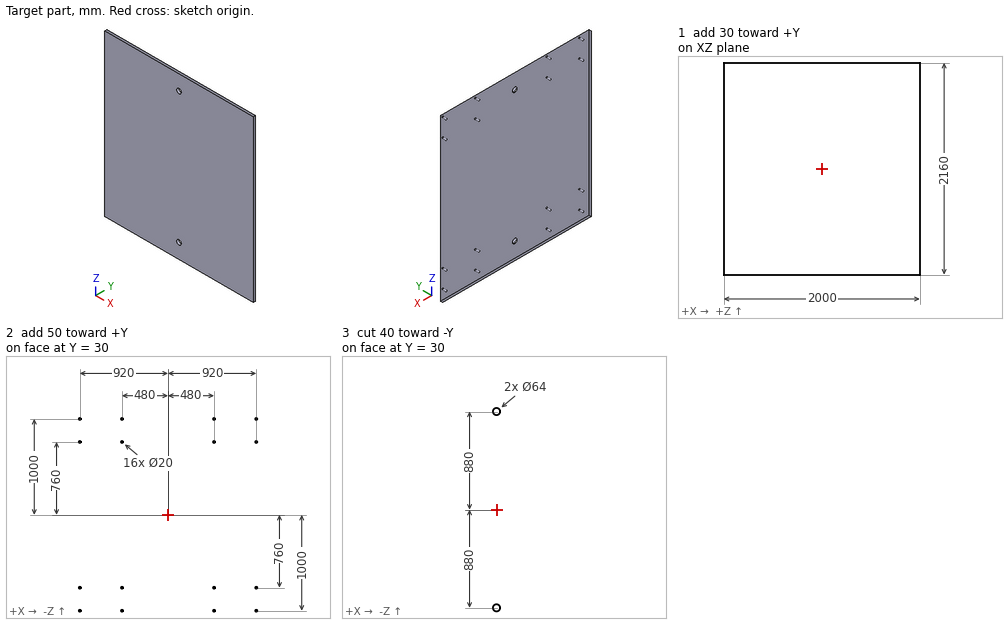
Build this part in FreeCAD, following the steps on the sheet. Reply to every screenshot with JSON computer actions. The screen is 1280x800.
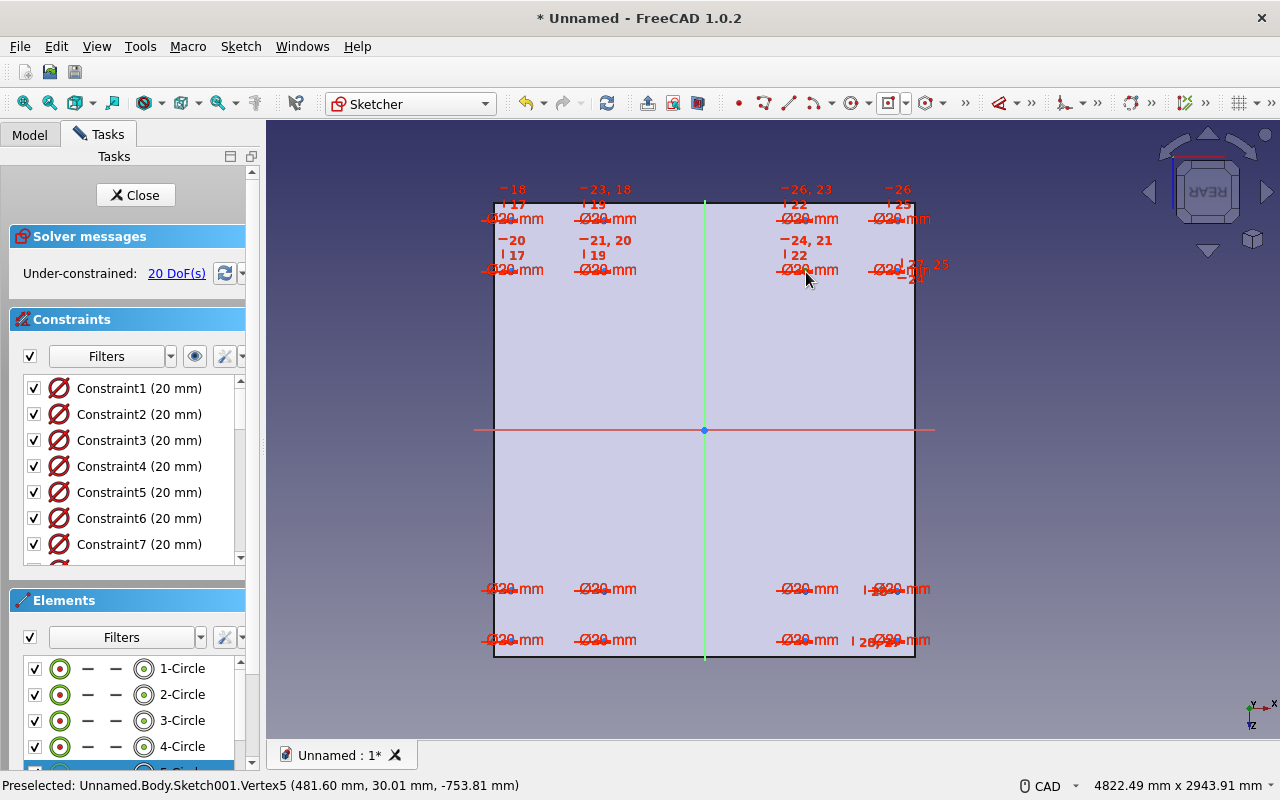
{"action": "left_click", "coordinate": [806, 642]}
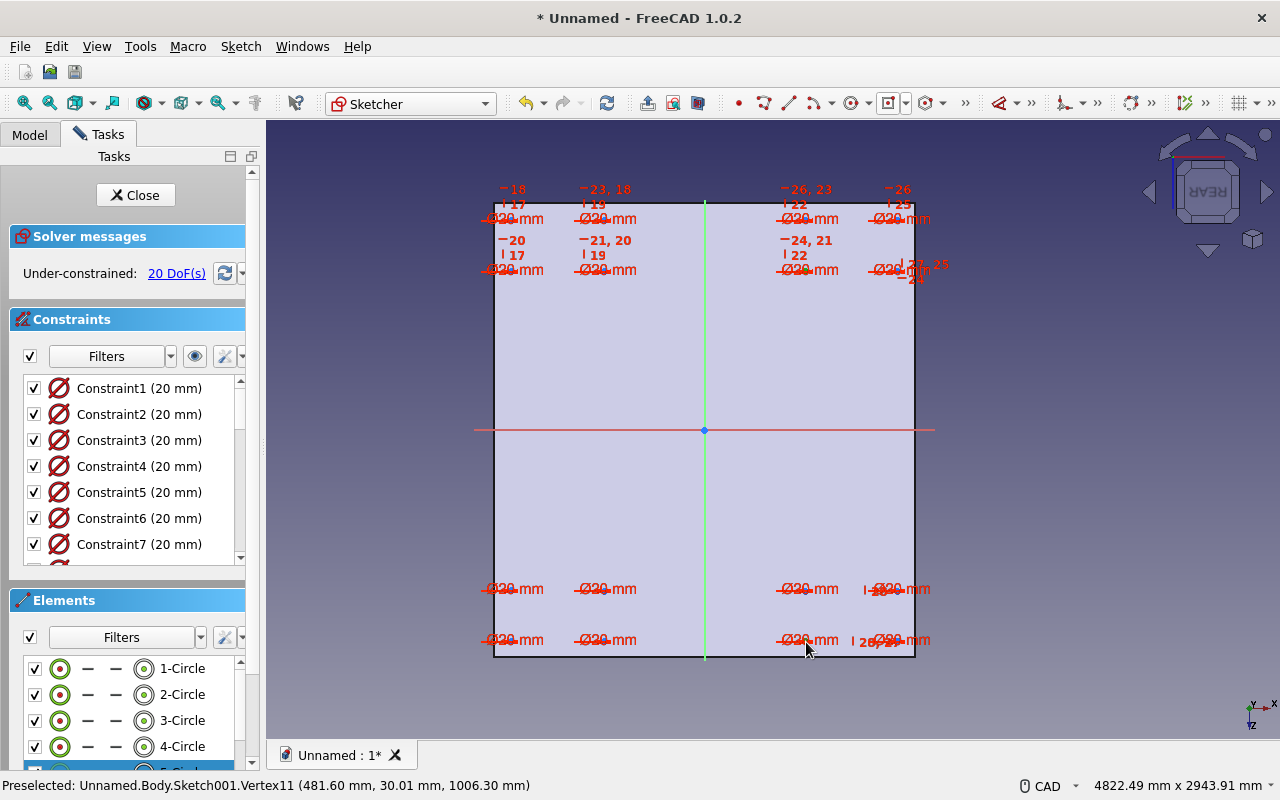
{"action": "key", "text": "v"}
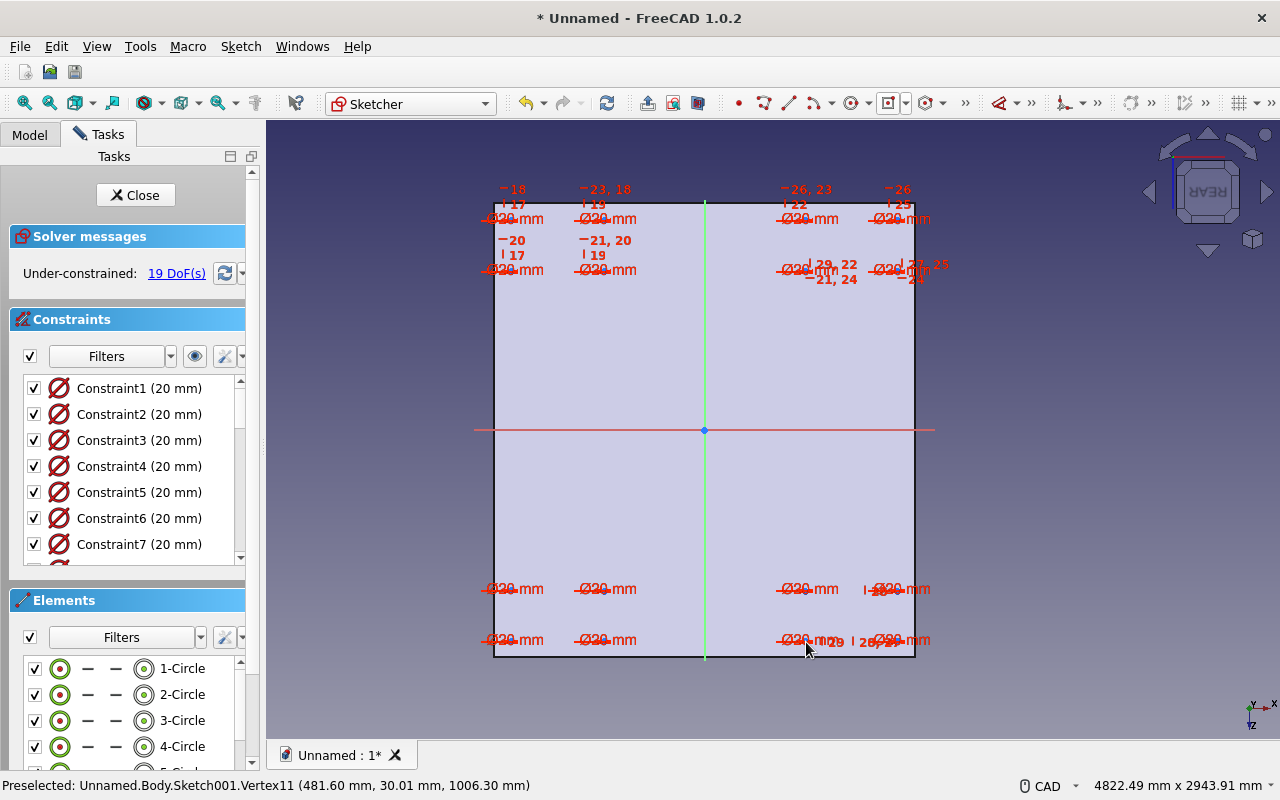
{"action": "left_click", "coordinate": [898, 642]}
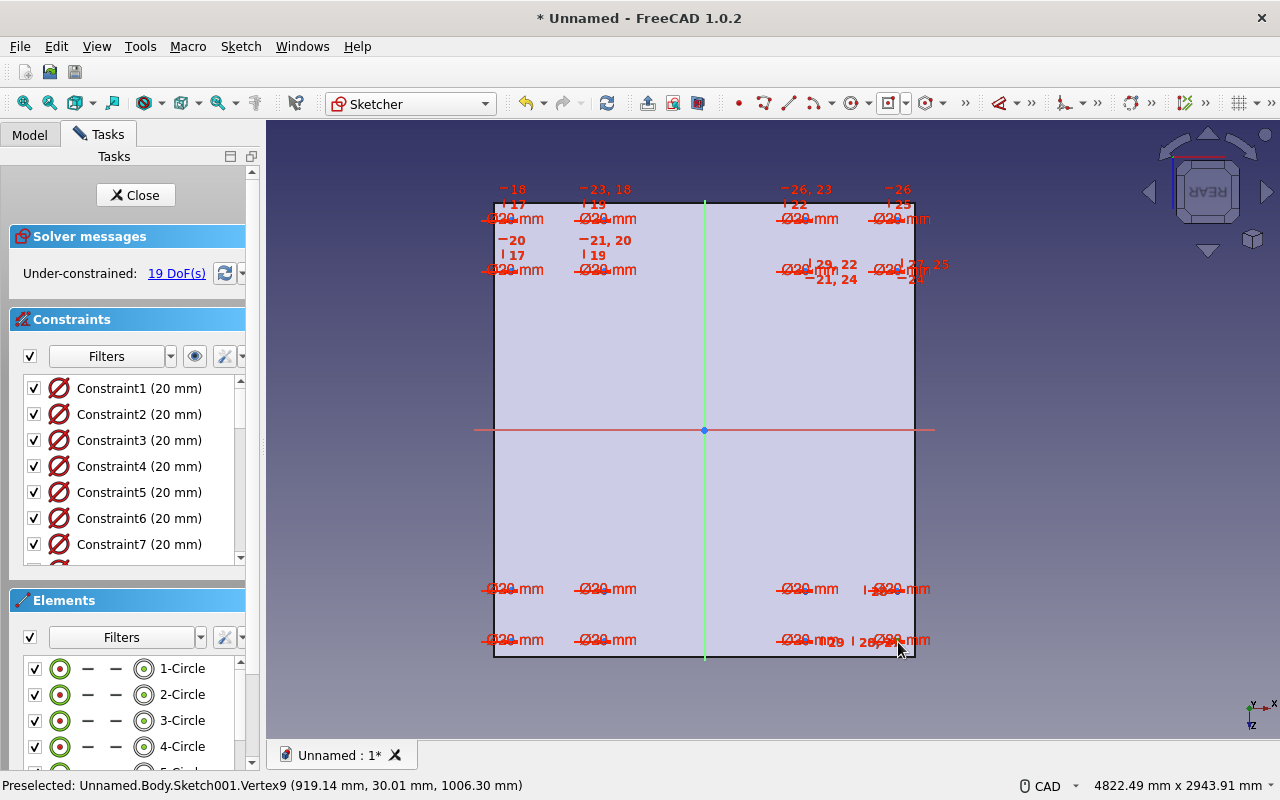
{"action": "left_click", "coordinate": [806, 642]}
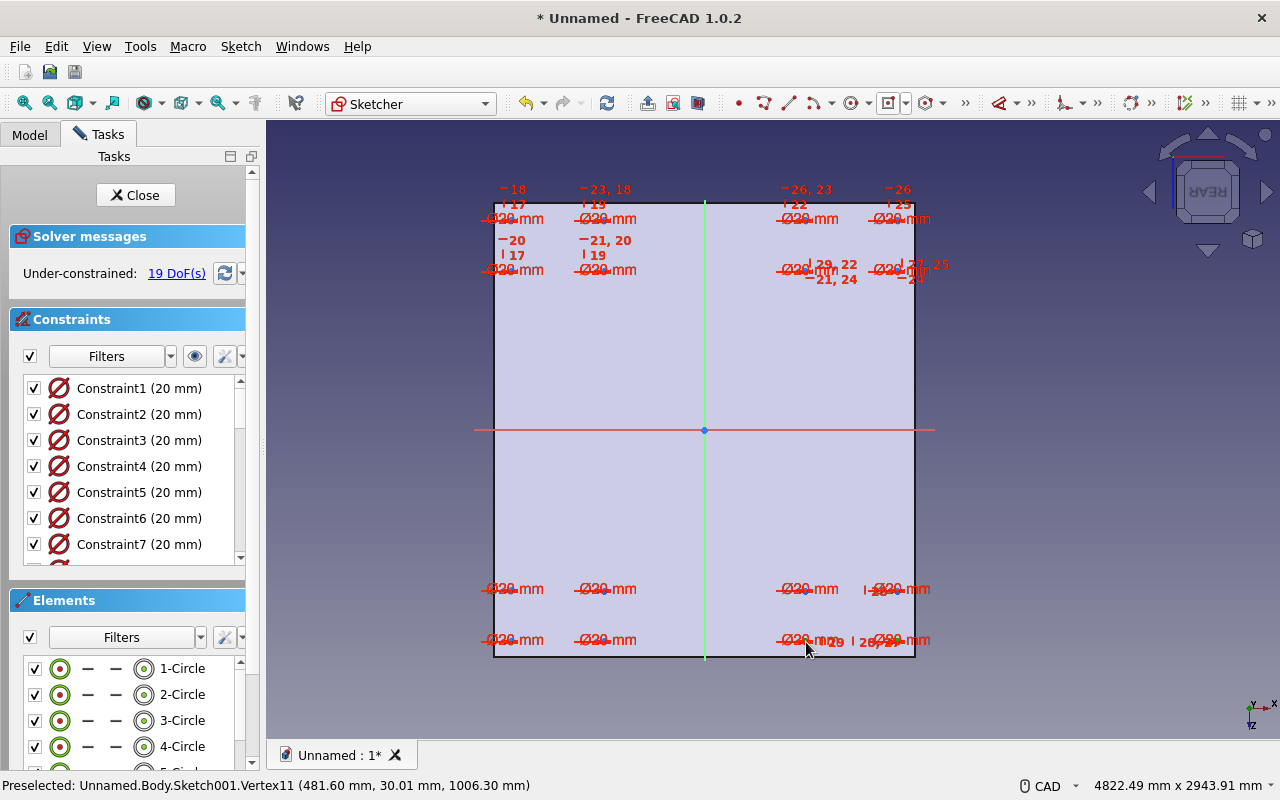
{"action": "key", "text": "h"}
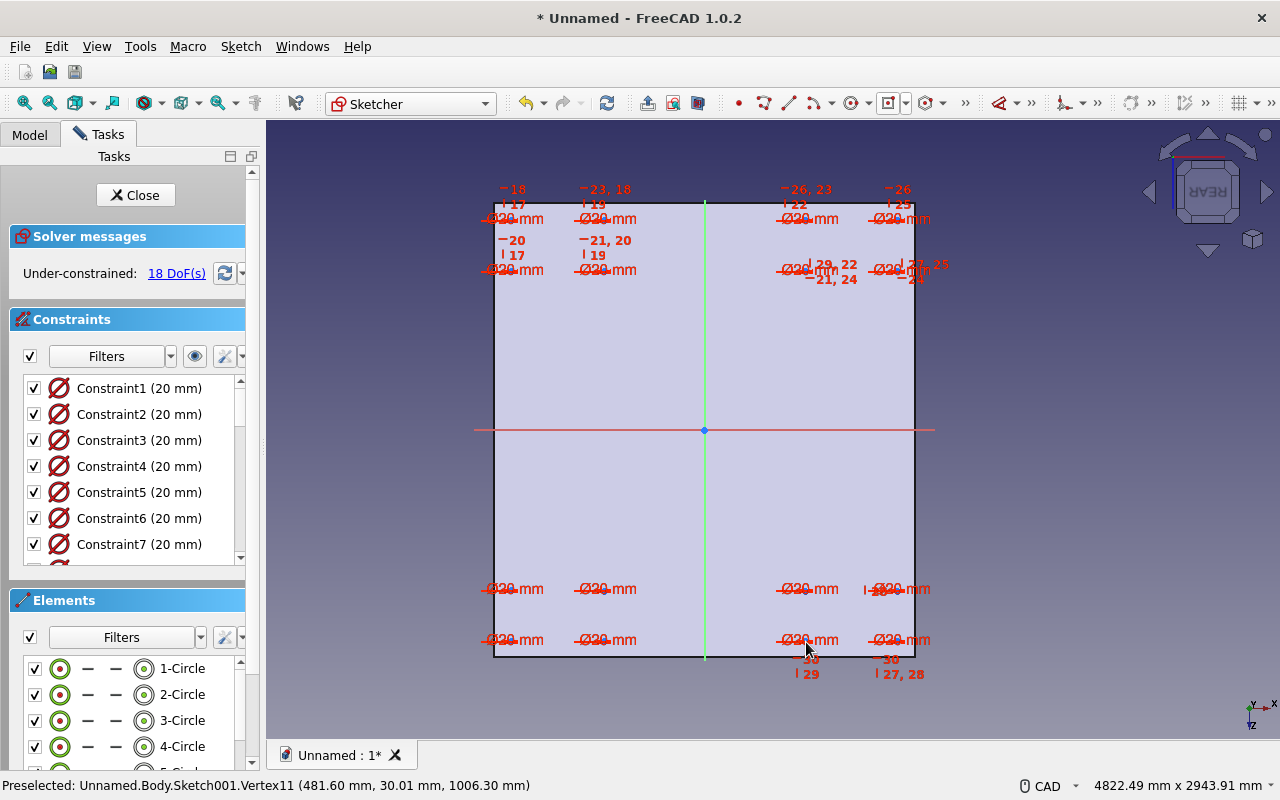
{"action": "left_click", "coordinate": [806, 642]}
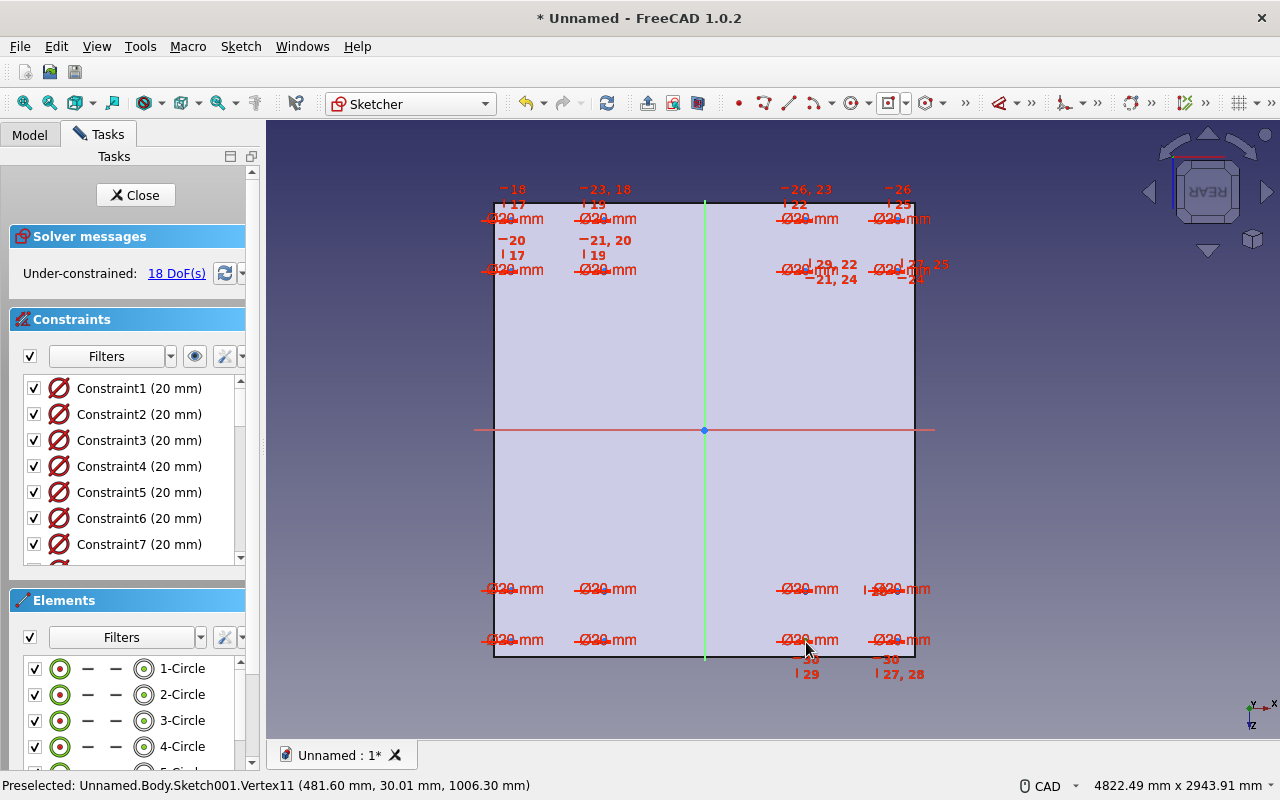
{"action": "left_click", "coordinate": [806, 591]}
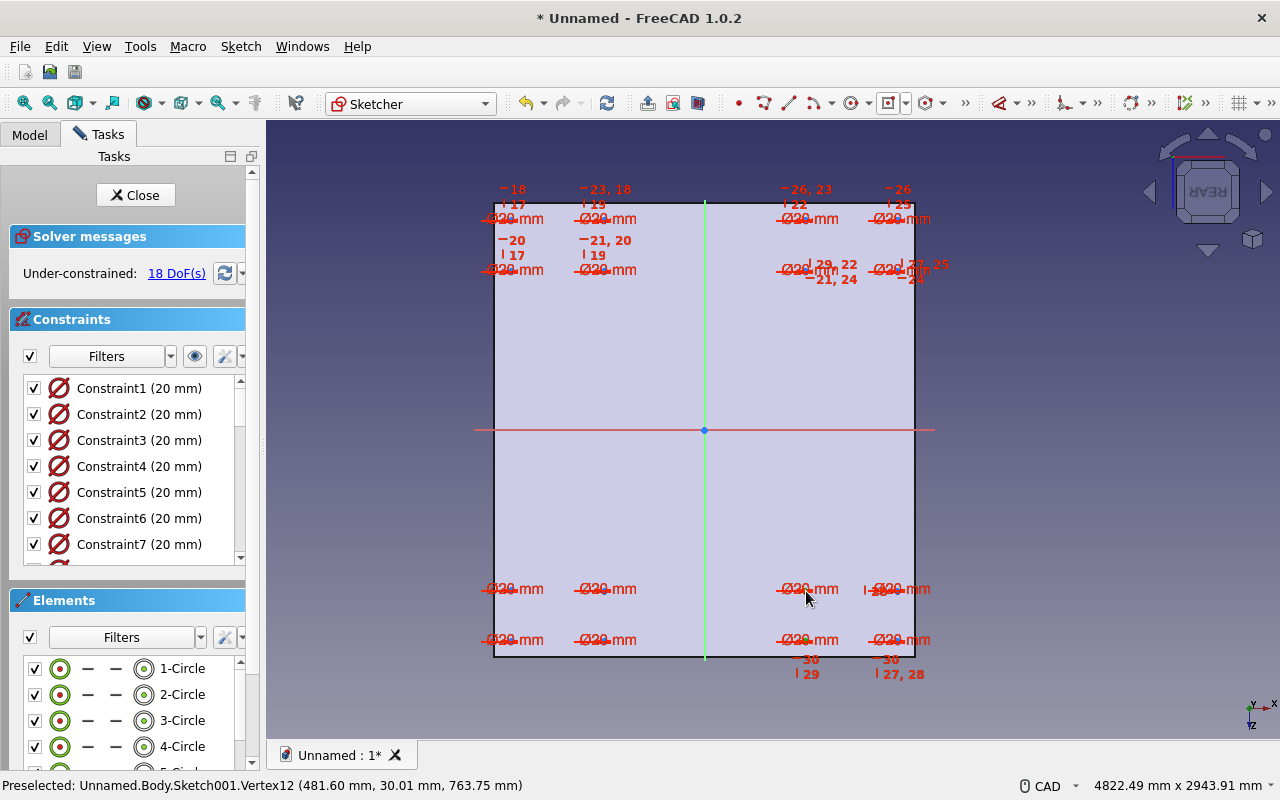
{"action": "key", "text": "v"}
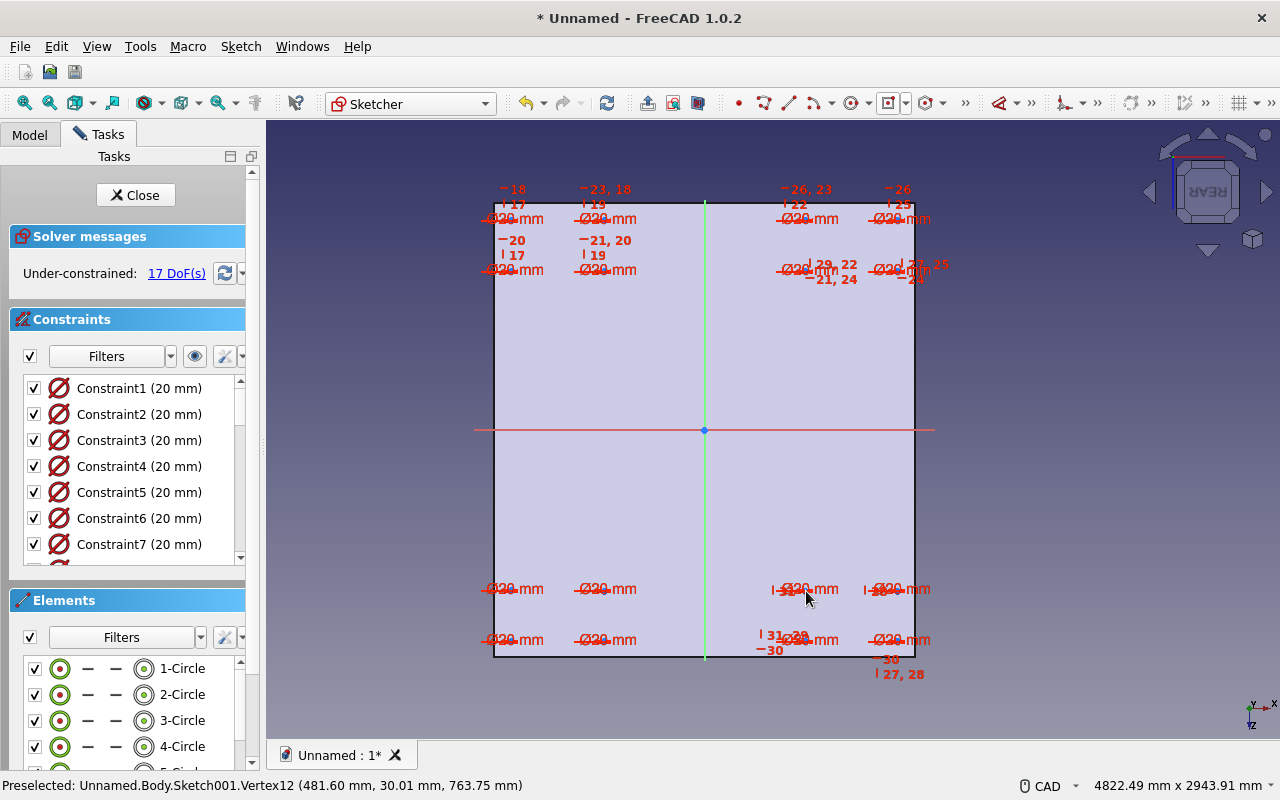
{"action": "left_click", "coordinate": [898, 591]}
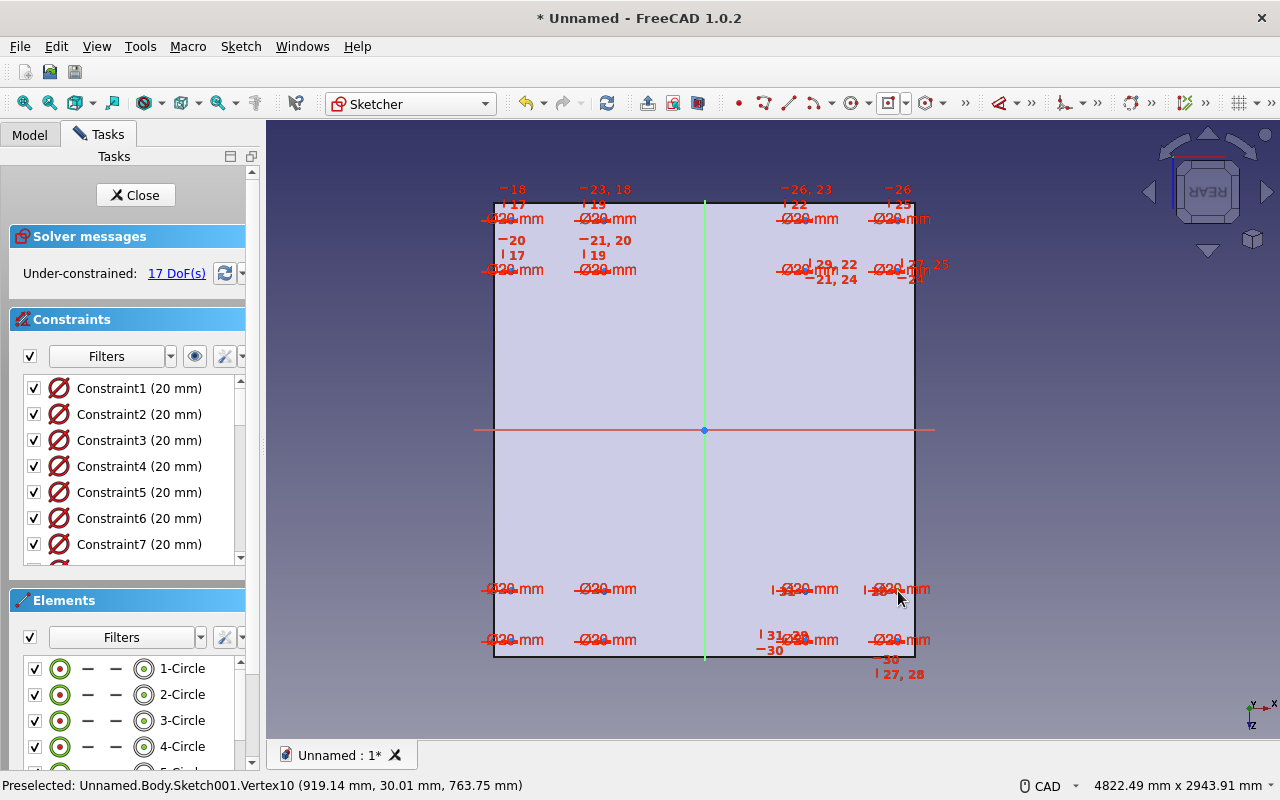
{"action": "left_click", "coordinate": [806, 591]}